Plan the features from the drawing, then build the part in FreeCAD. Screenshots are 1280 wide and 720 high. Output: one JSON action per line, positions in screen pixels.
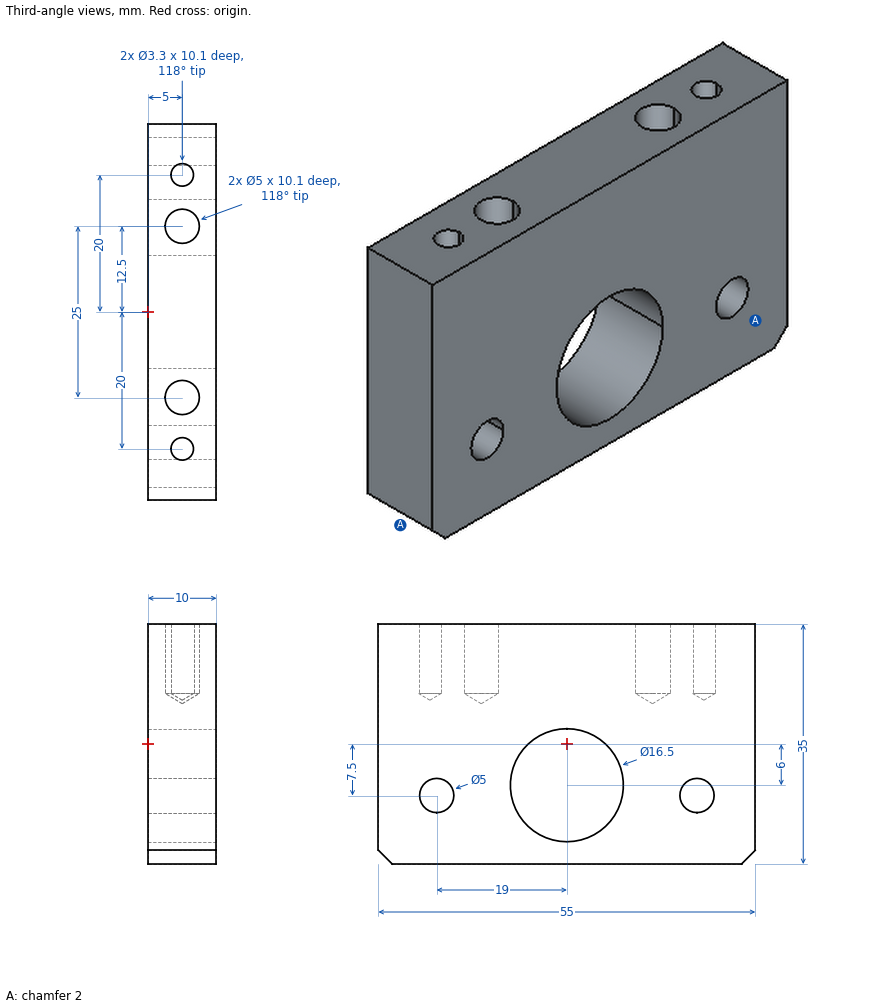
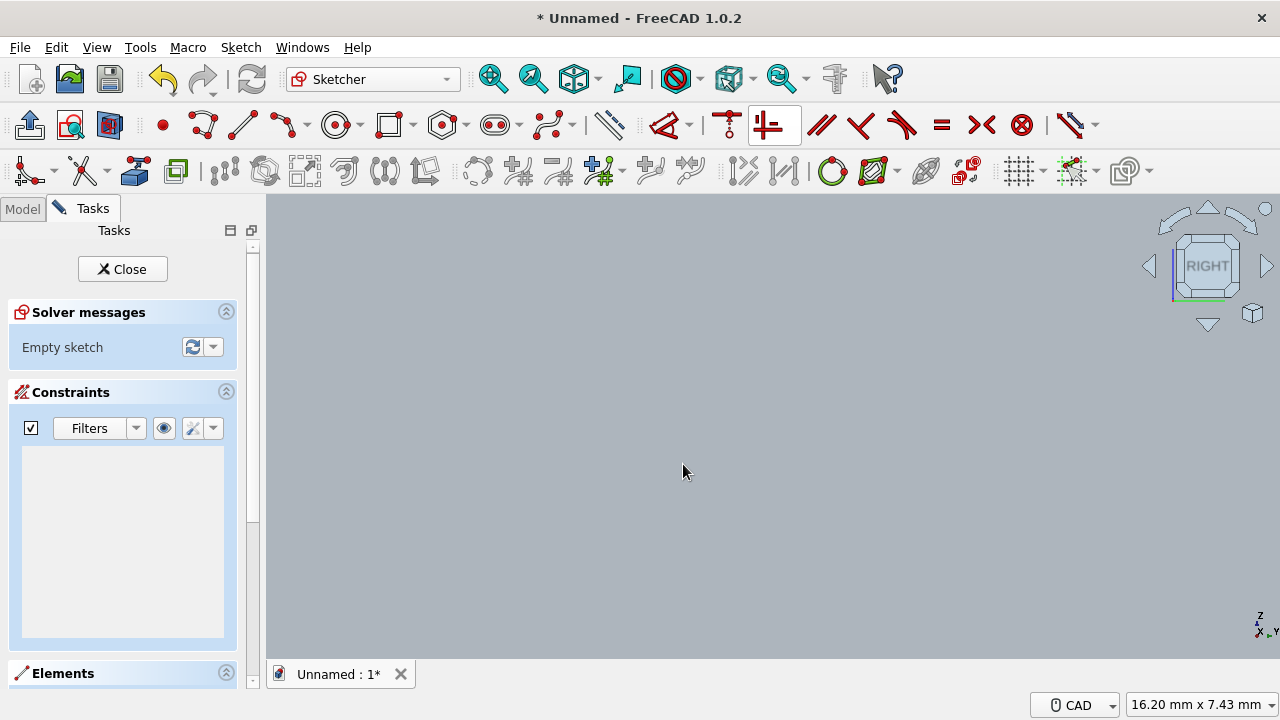
{"action": "left_click", "coordinate": [336, 126]}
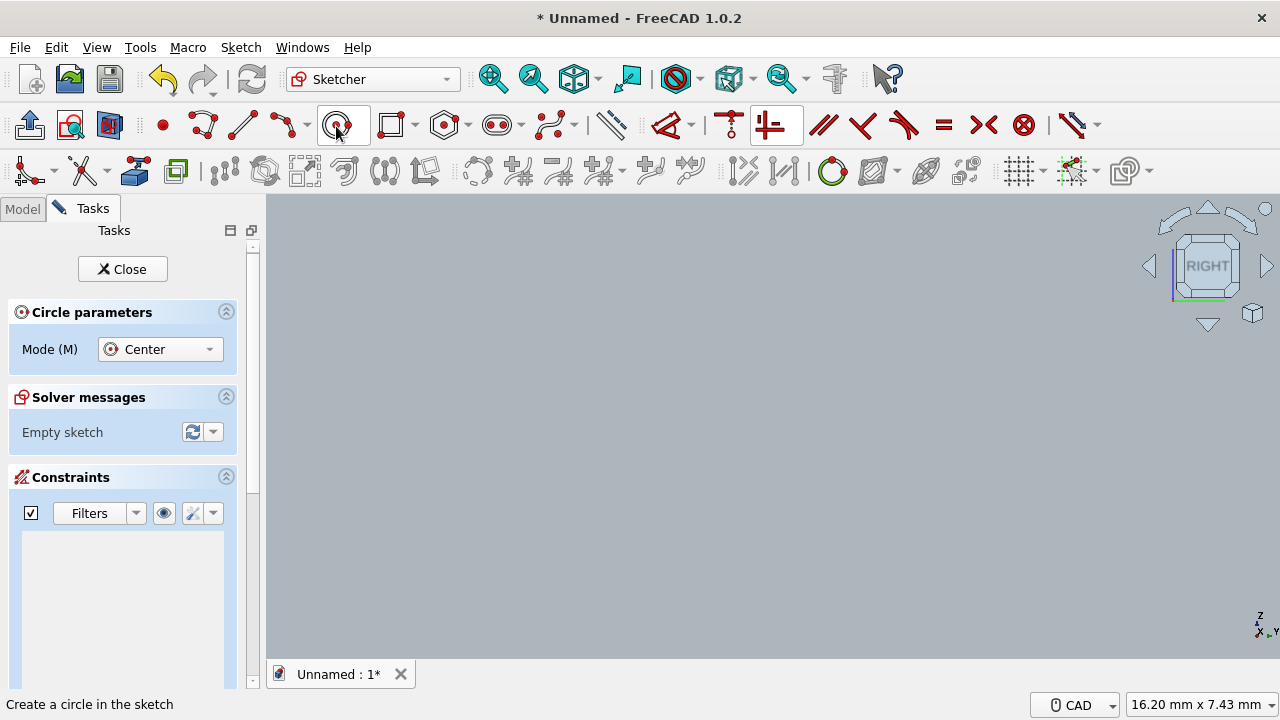
{"action": "left_click", "coordinate": [700, 421]}
{"action": "mouse_move", "coordinate": [811, 311]}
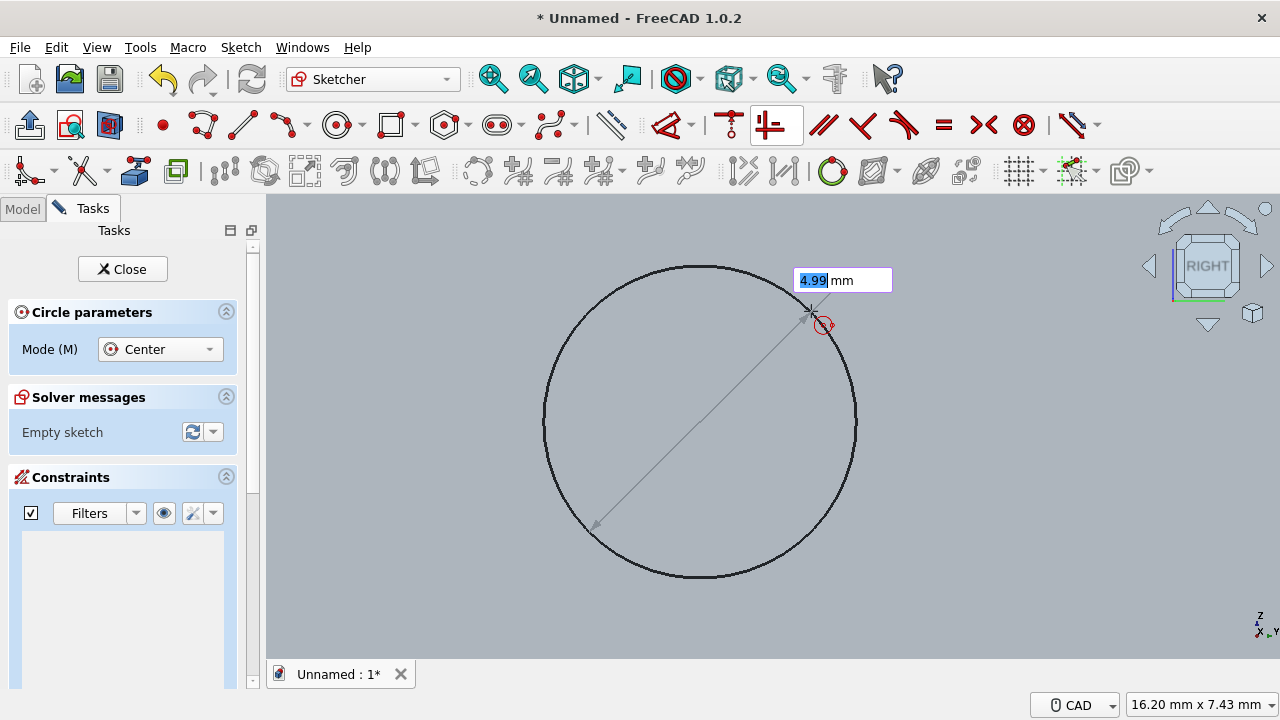
{"action": "type", "text": "5"}
{"action": "key", "text": "Return"}
{"action": "key", "text": "Escape"}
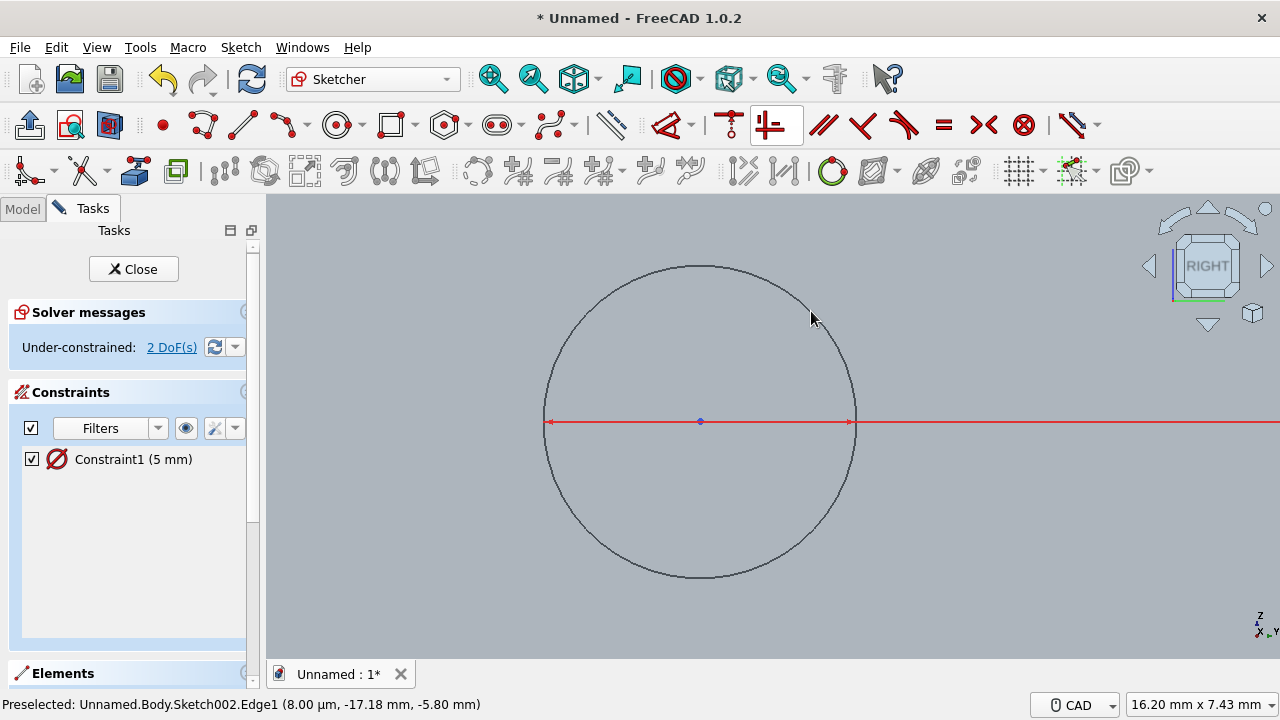
{"action": "left_click", "coordinate": [666, 126]}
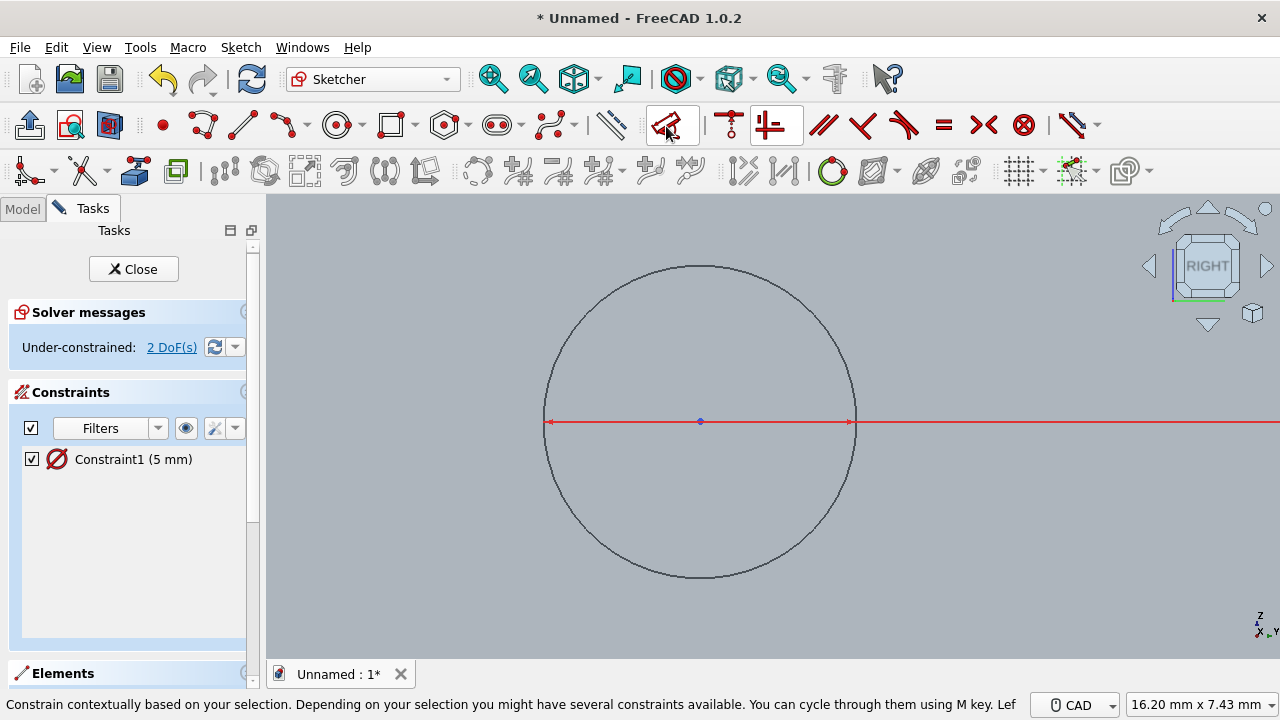
{"action": "left_click", "coordinate": [700, 422]}
{"action": "left_click", "coordinate": [907, 456]}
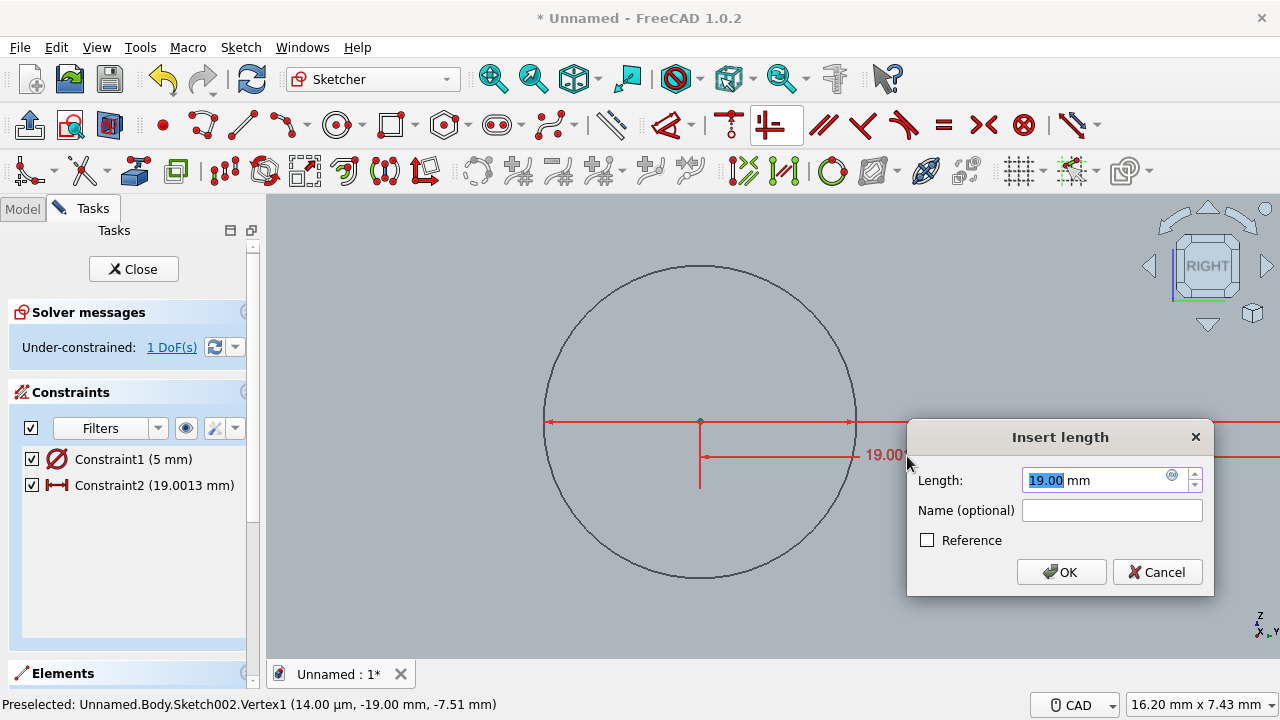
{"action": "type", "text": "19"}
{"action": "key", "text": "Return"}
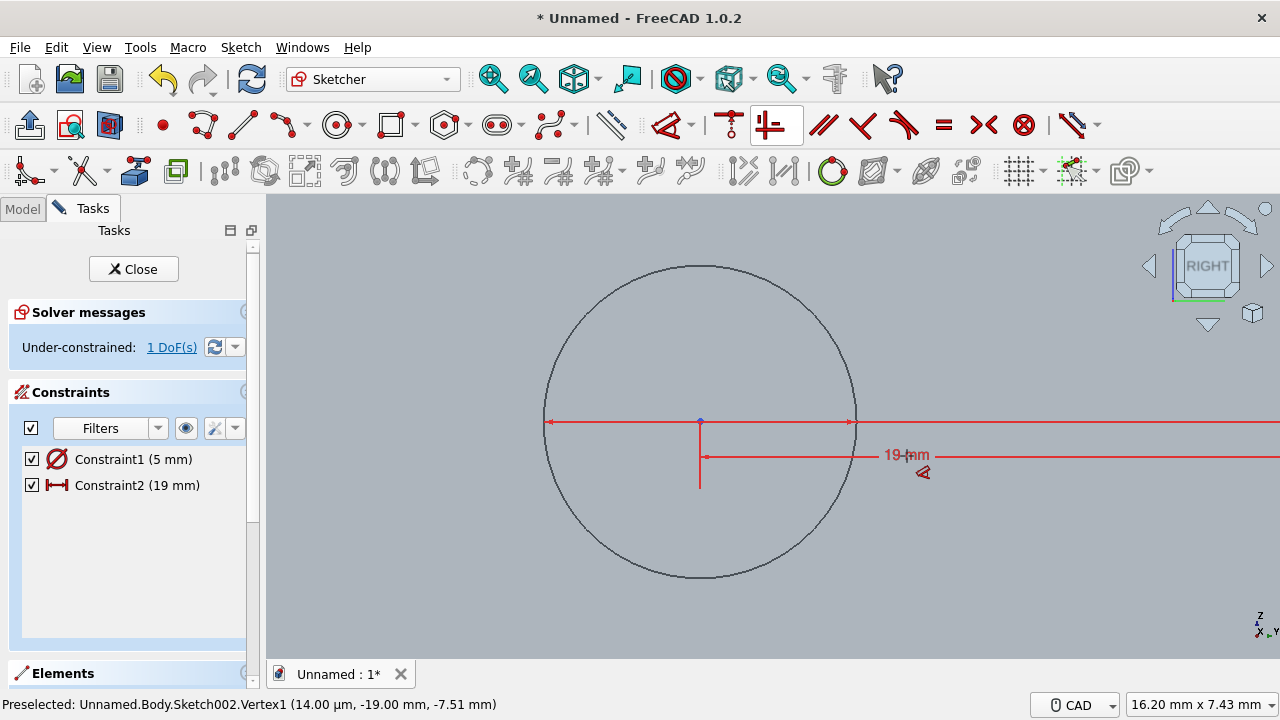
{"action": "left_click", "coordinate": [700, 422]}
{"action": "left_click", "coordinate": [666, 322]}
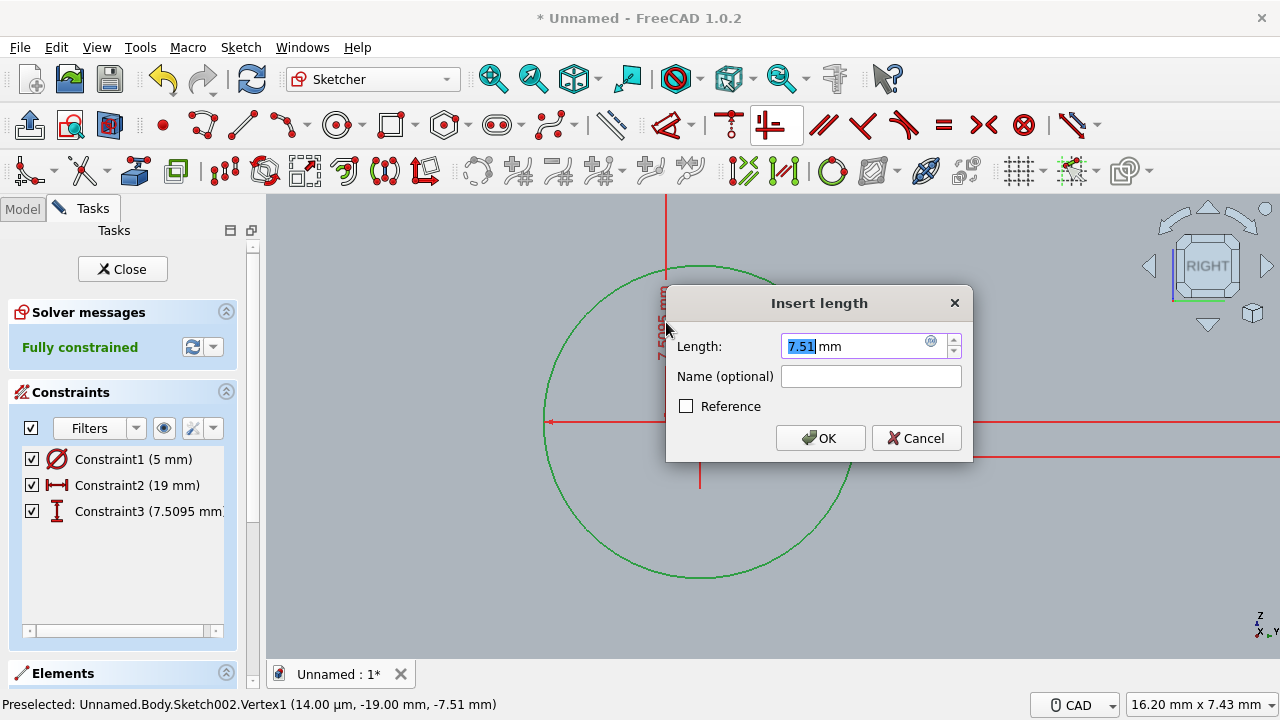
{"action": "type", "text": "7.5"}
{"action": "key", "text": "Return"}
{"action": "key", "text": "Escape"}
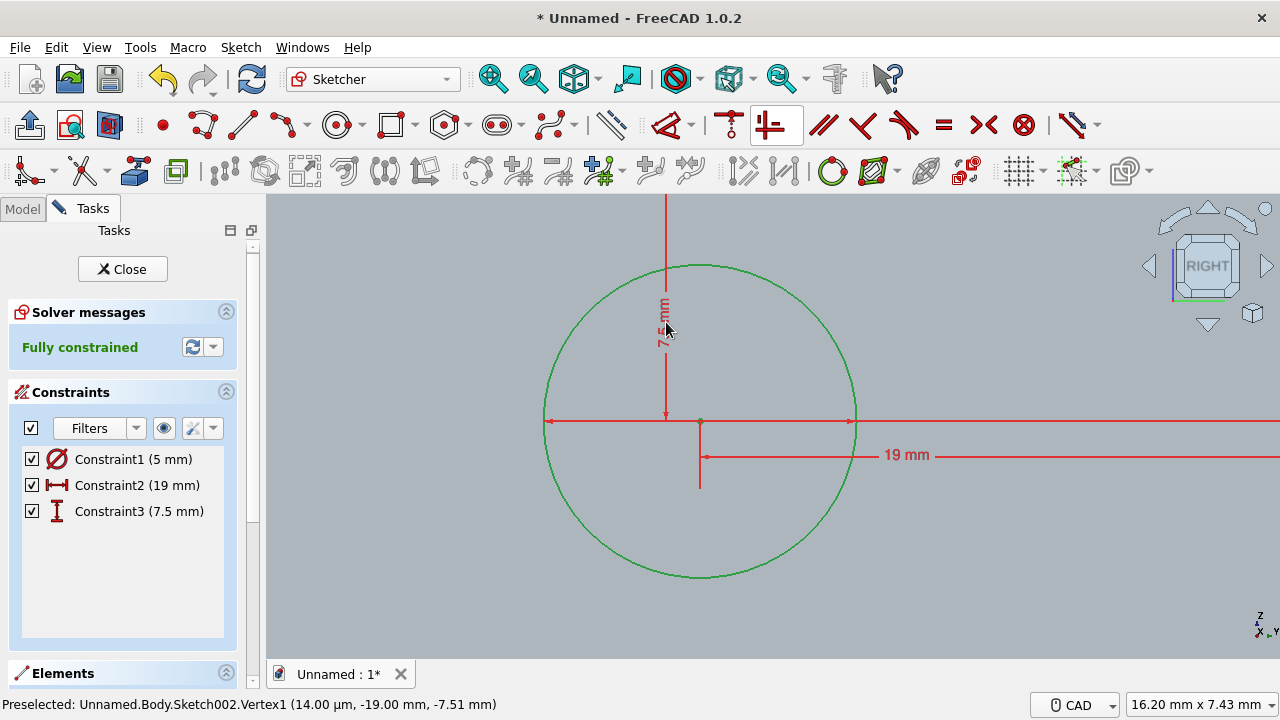
{"action": "left_click", "coordinate": [123, 269]}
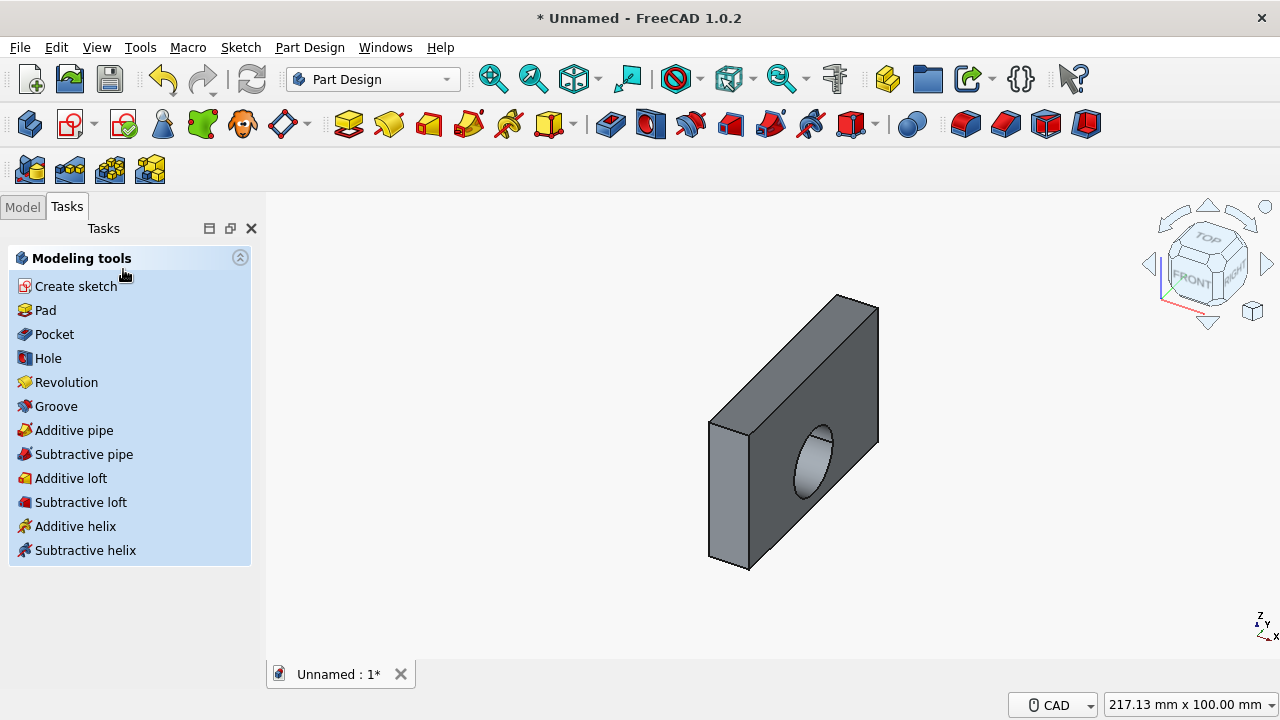
{"action": "left_click", "coordinate": [612, 124]}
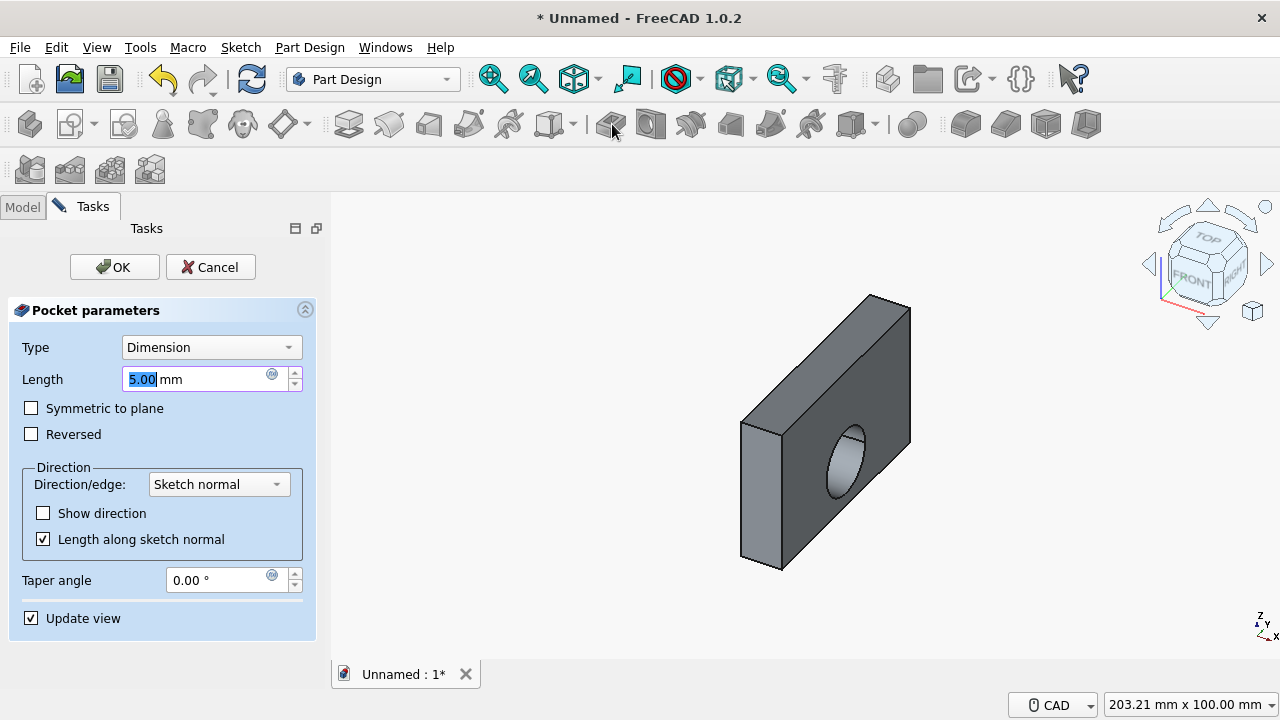
{"action": "left_click", "coordinate": [212, 348]}